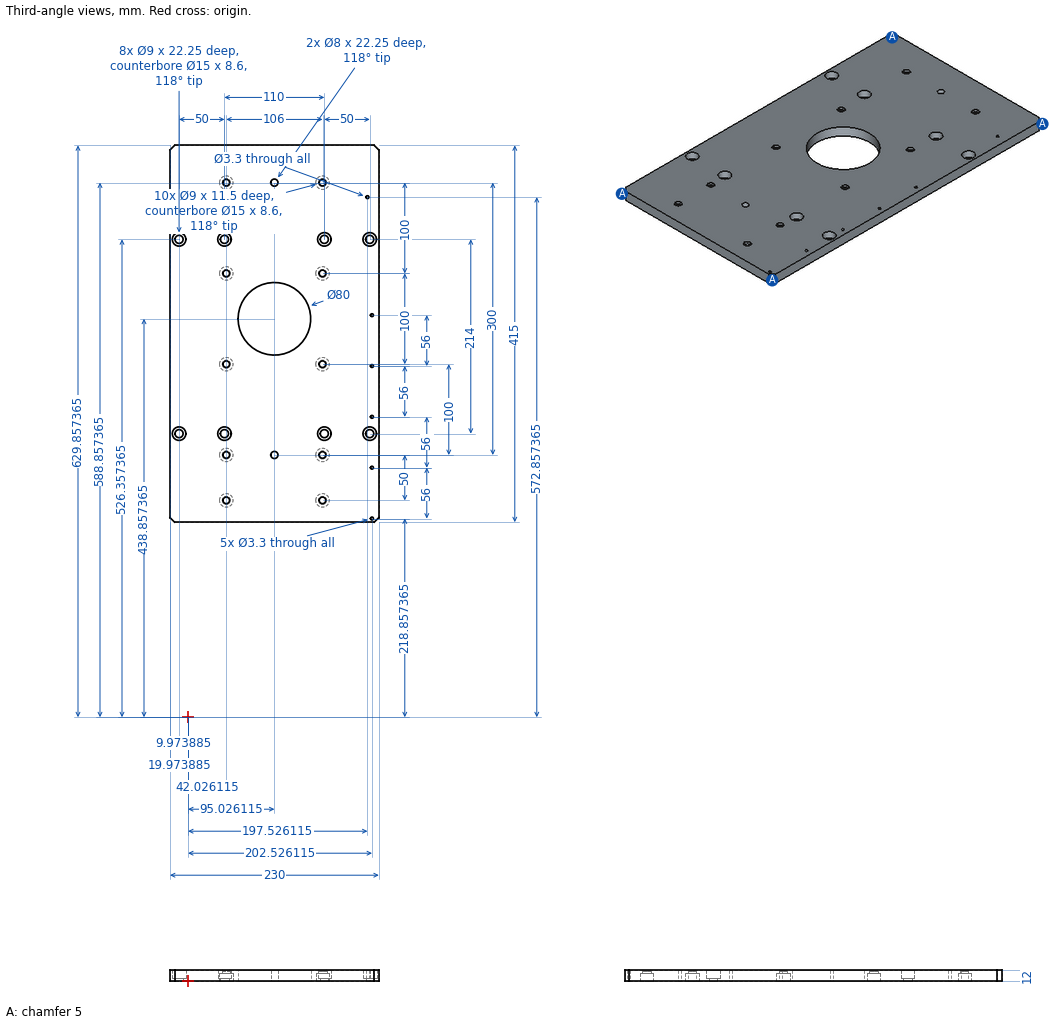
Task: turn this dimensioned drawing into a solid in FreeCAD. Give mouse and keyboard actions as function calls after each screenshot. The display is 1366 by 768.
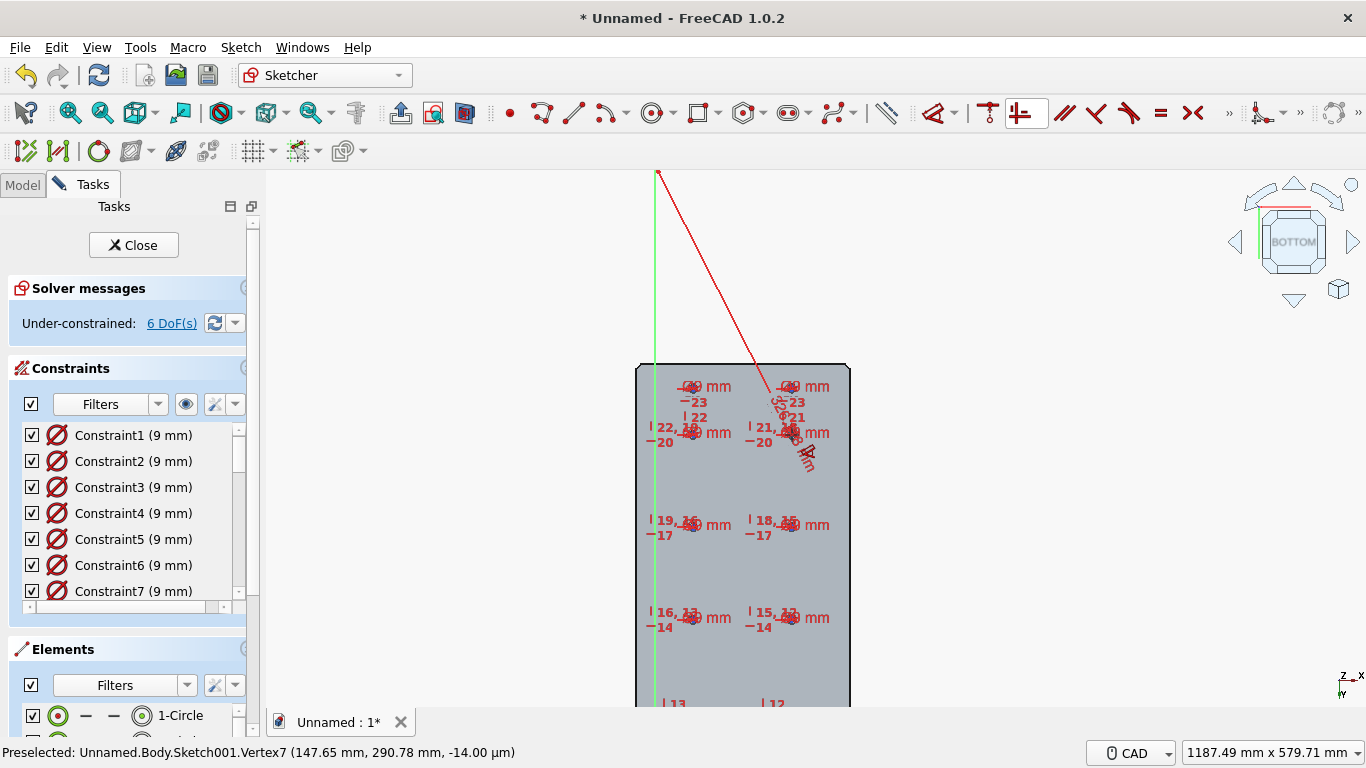
click(792, 389)
click(826, 412)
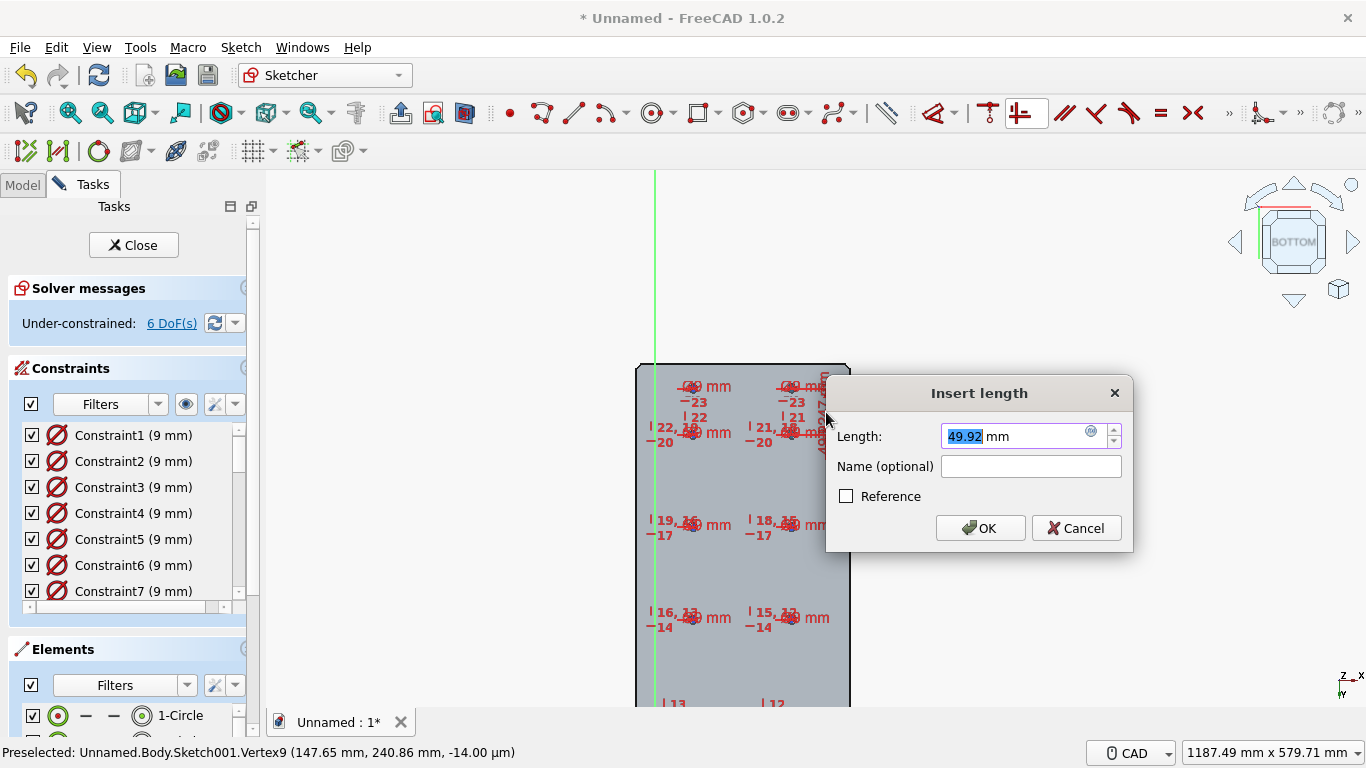
text(50)
key(Return)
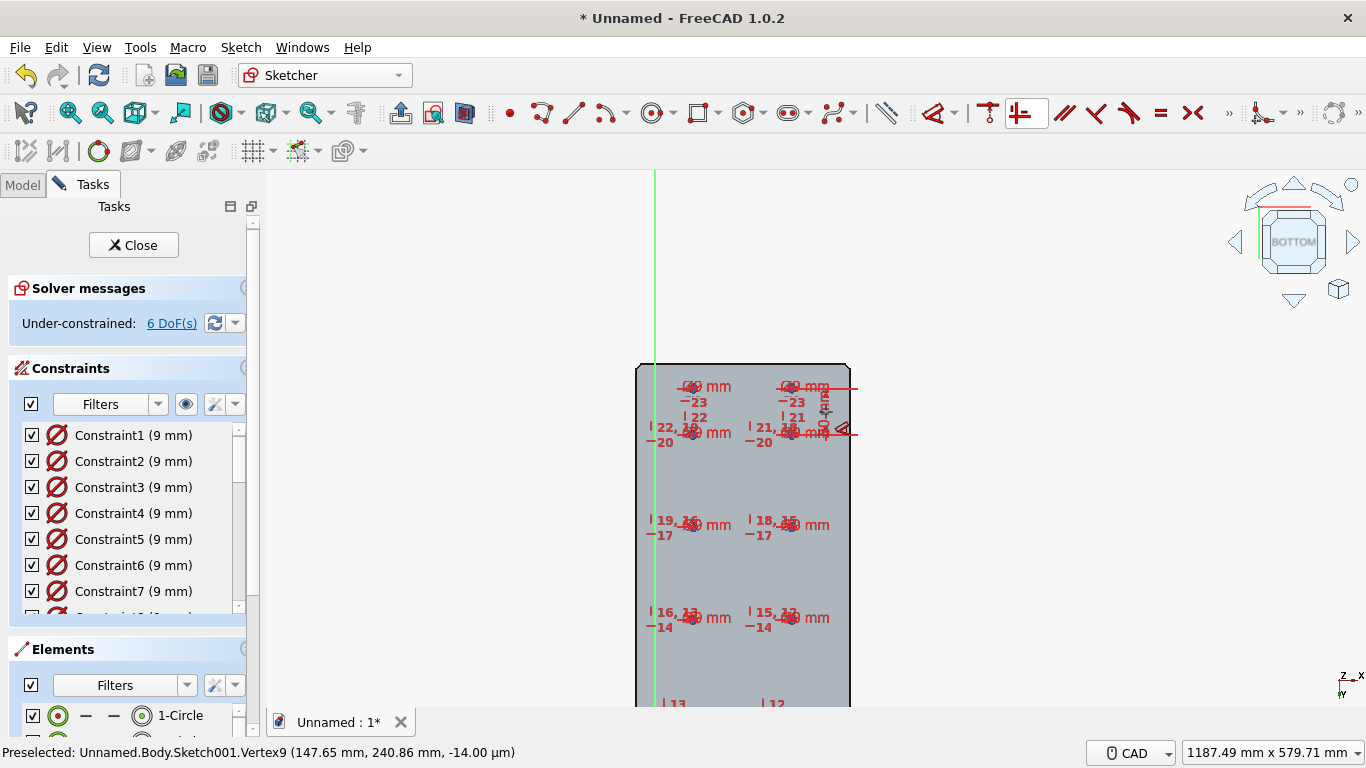
scroll(792, 435, down, 2)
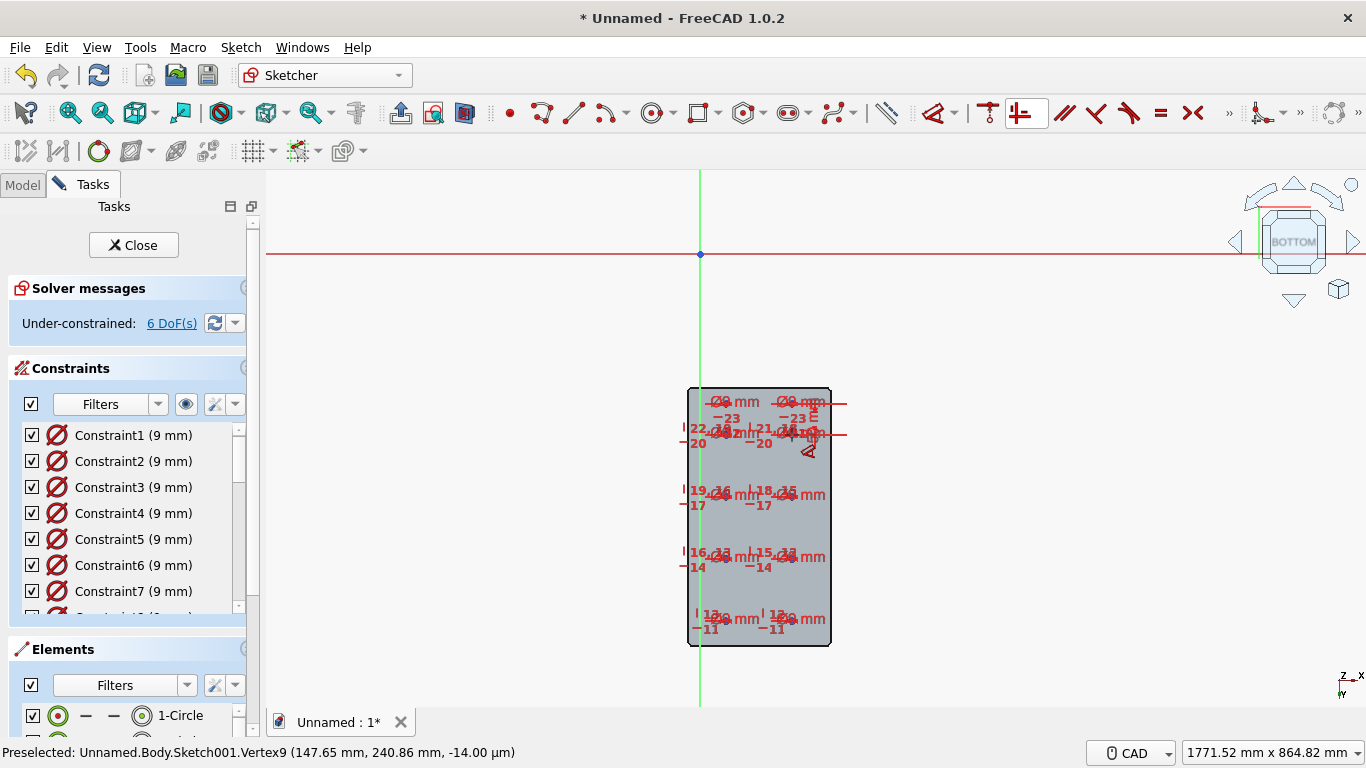
click(792, 621)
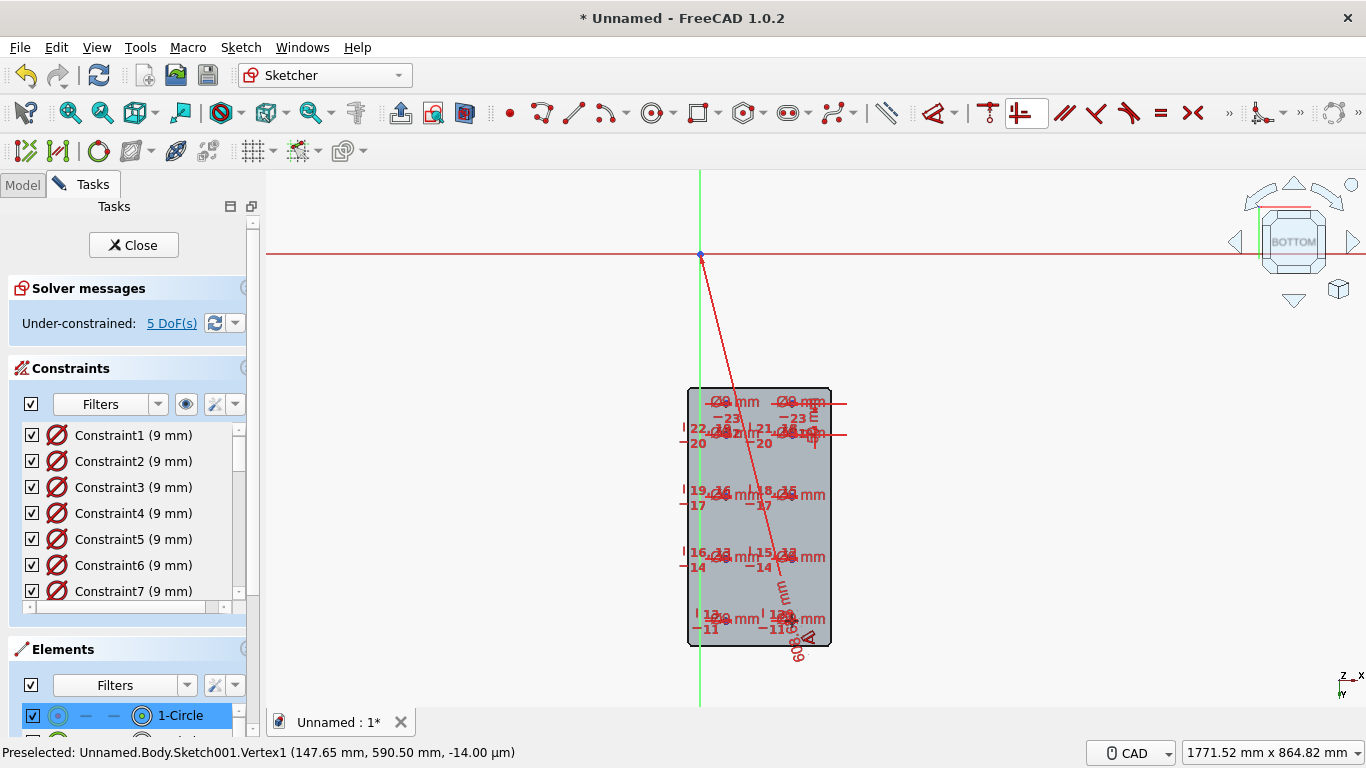
click(726, 621)
click(759, 655)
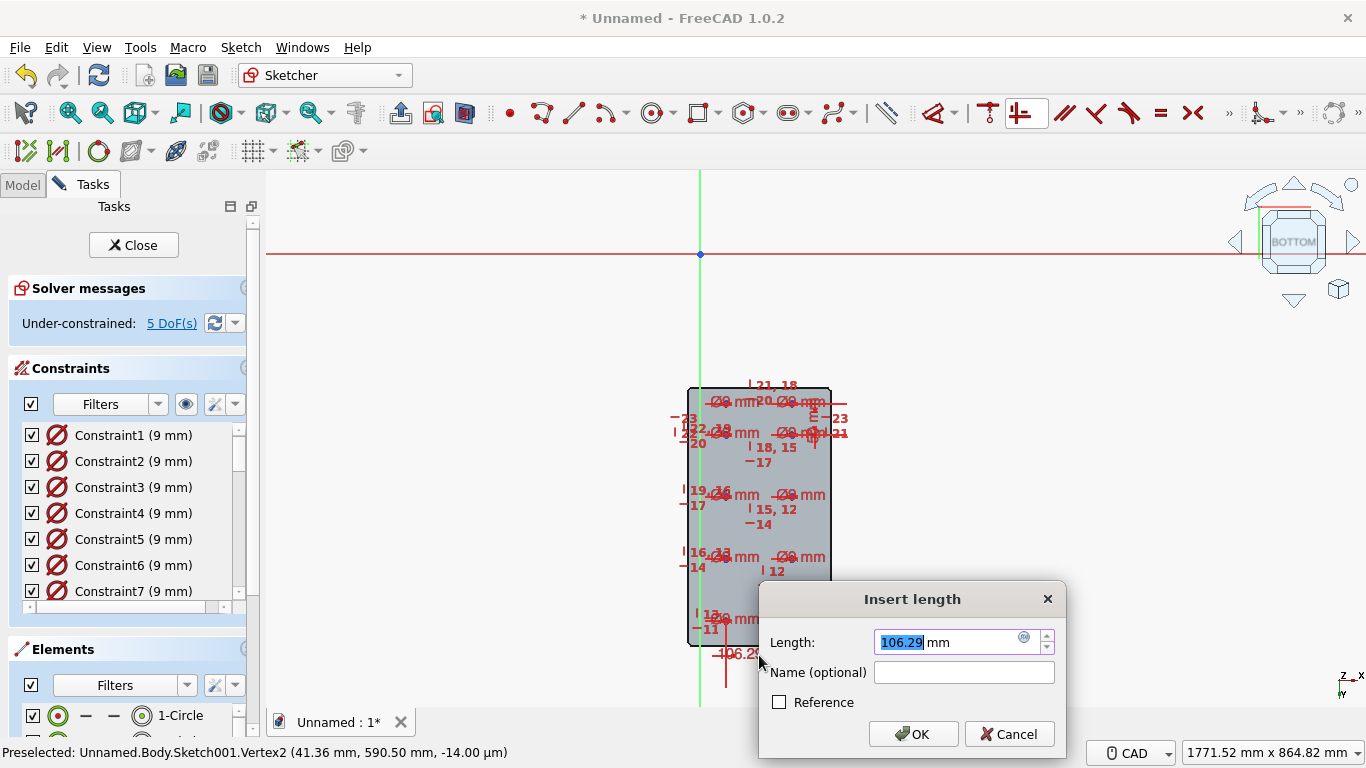
text(106)
key(Return)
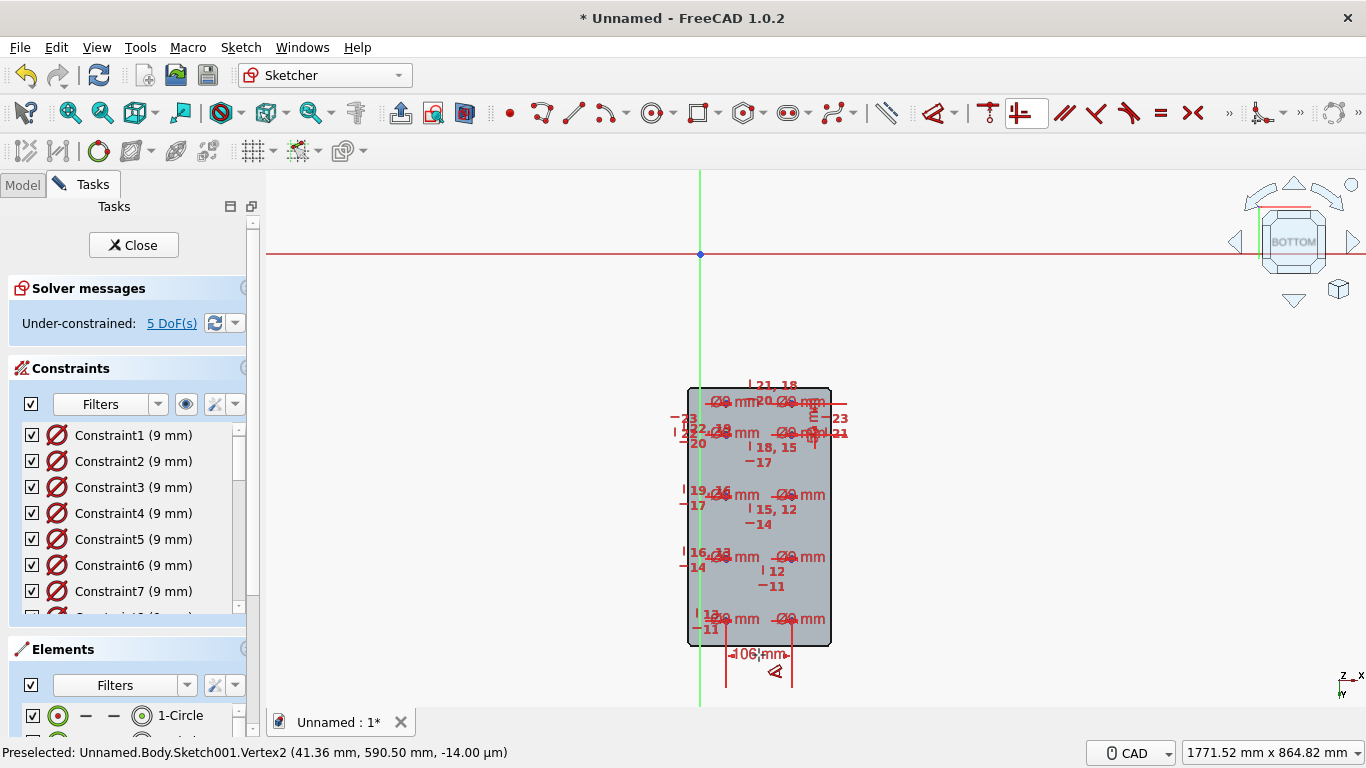
click(792, 621)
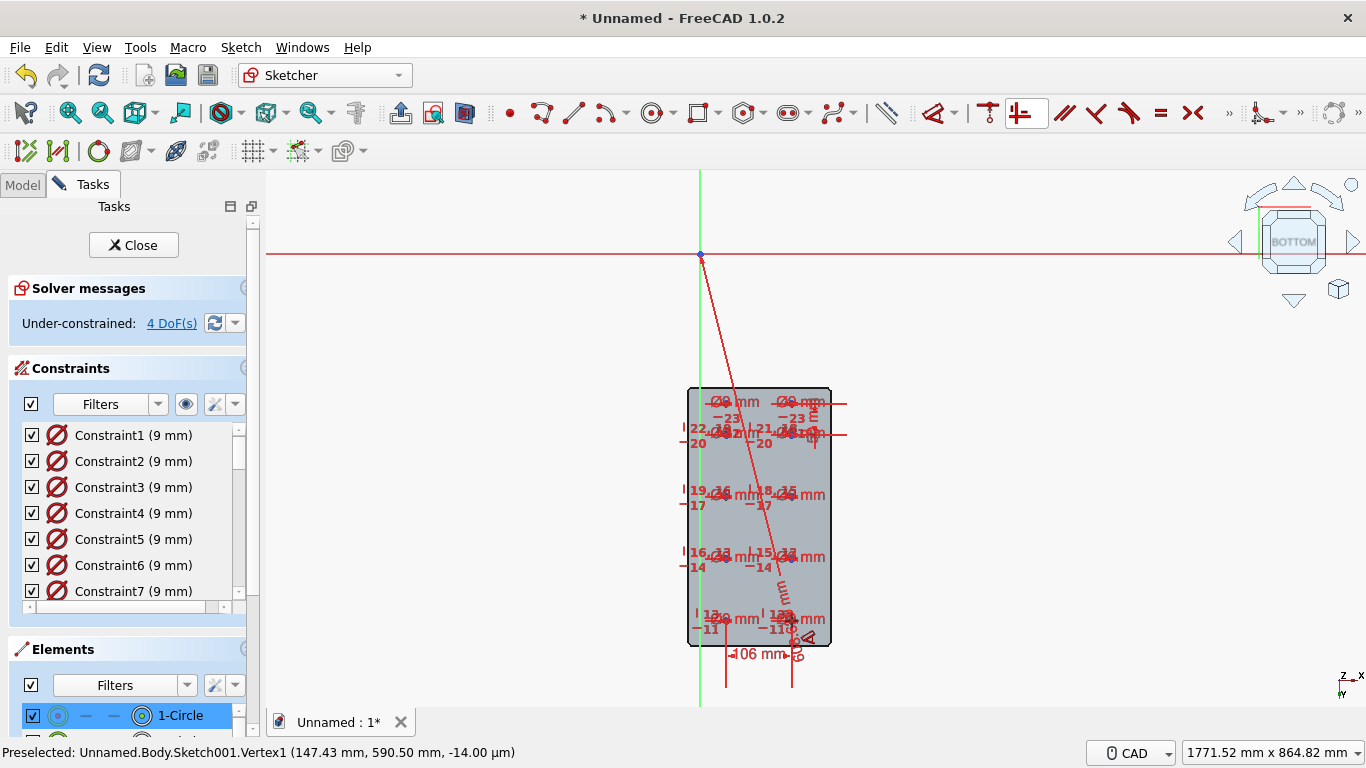
click(792, 559)
click(826, 590)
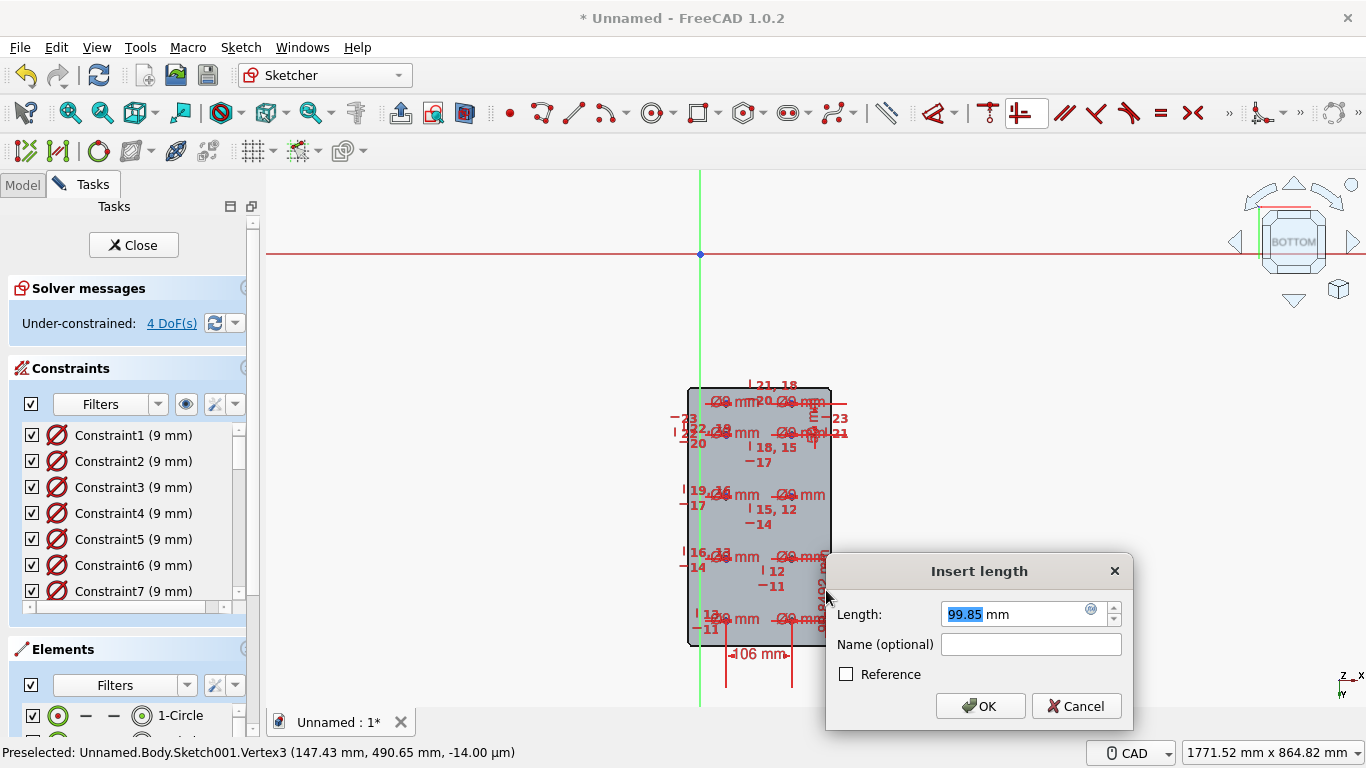
text(100)
key(Return)